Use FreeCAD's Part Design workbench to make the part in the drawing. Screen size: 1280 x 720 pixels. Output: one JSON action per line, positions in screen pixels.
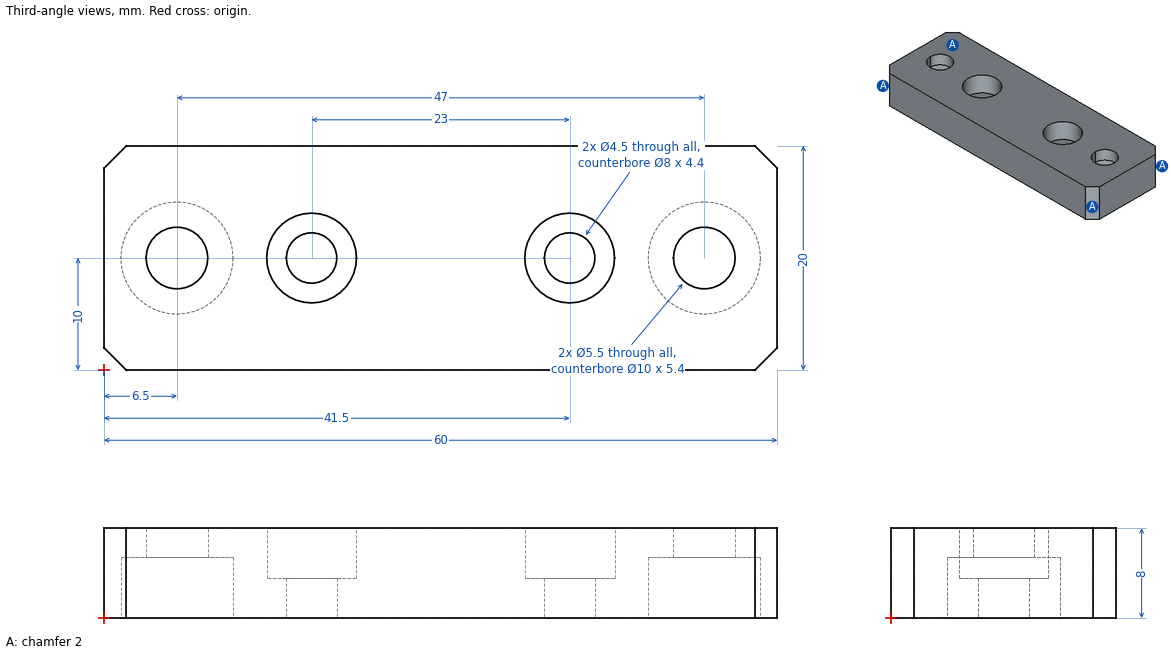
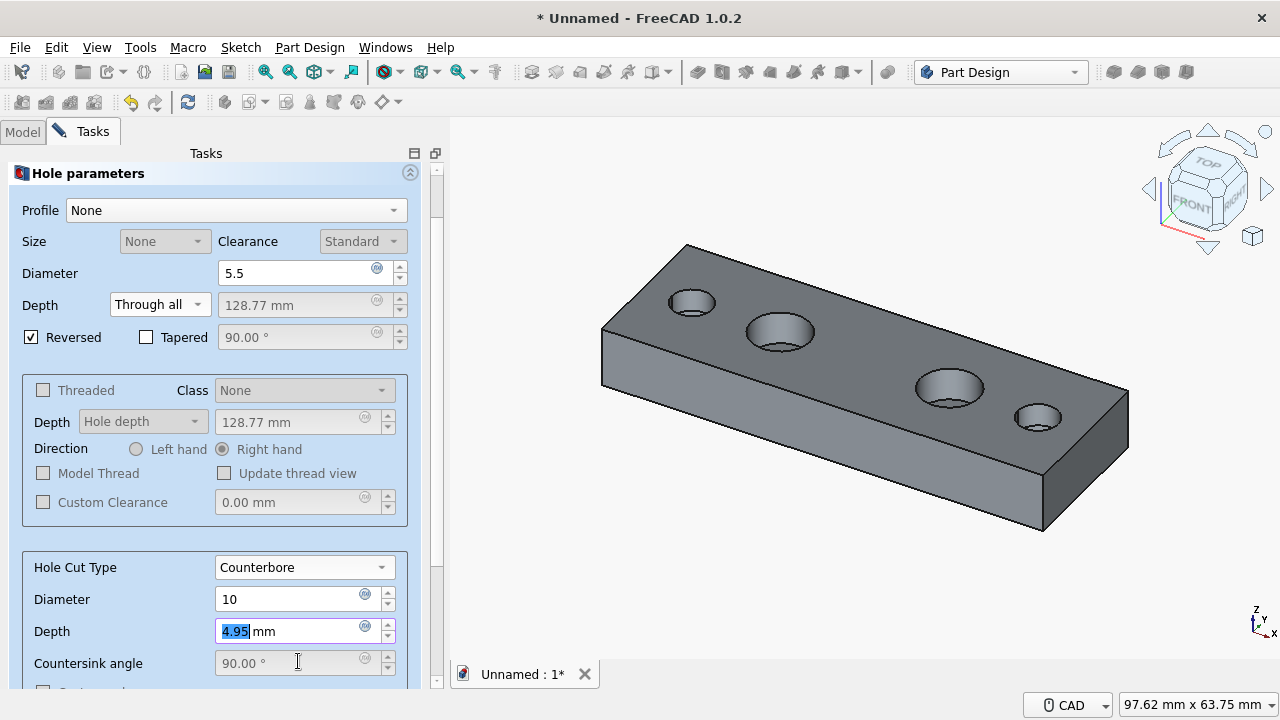
{"action": "type", "text": "5.4"}
{"action": "key", "text": "Tab"}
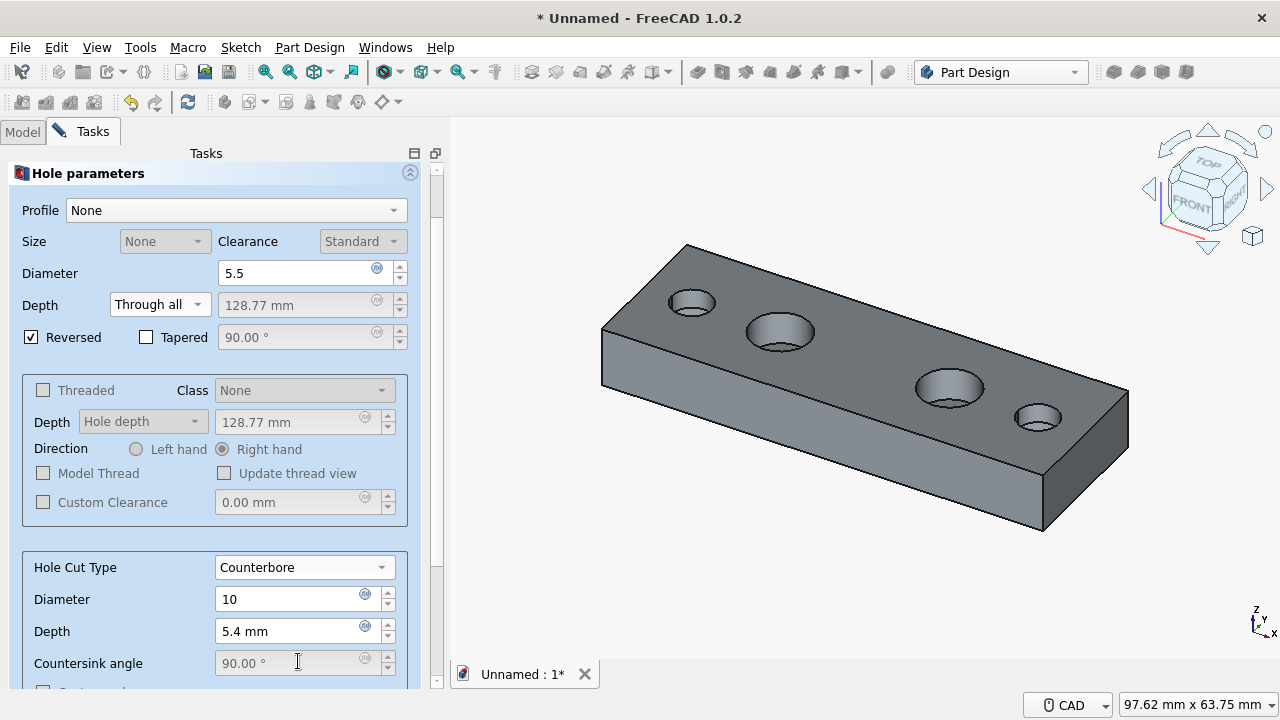
{"action": "scroll", "coordinate": [437, 426], "scroll_direction": "up", "scroll_amount": 2}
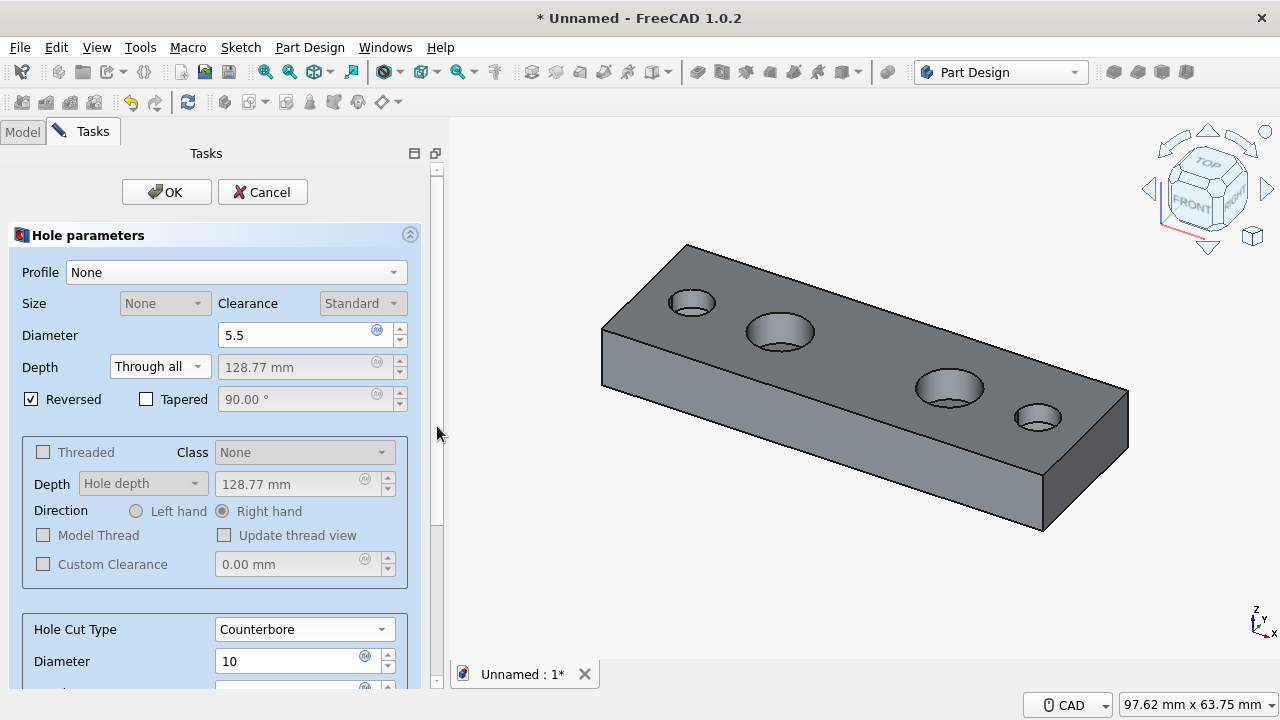
{"action": "left_click", "coordinate": [167, 192]}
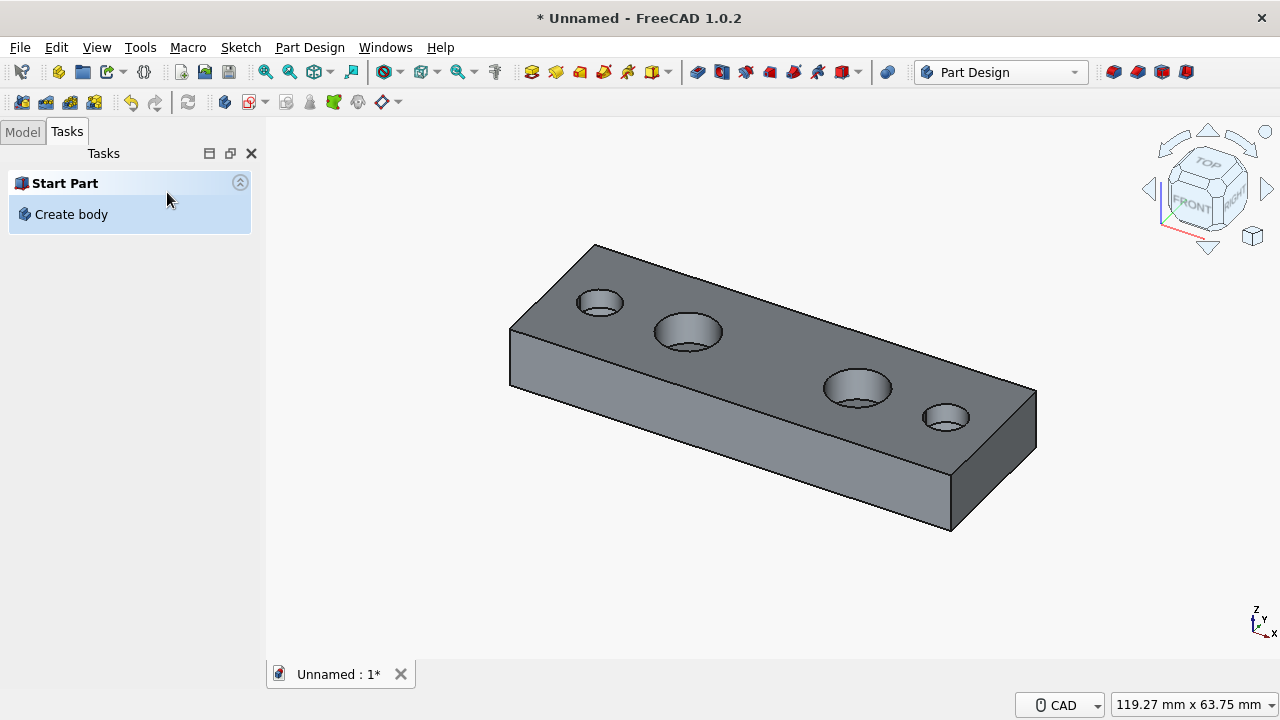
{"action": "left_click", "coordinate": [951, 502]}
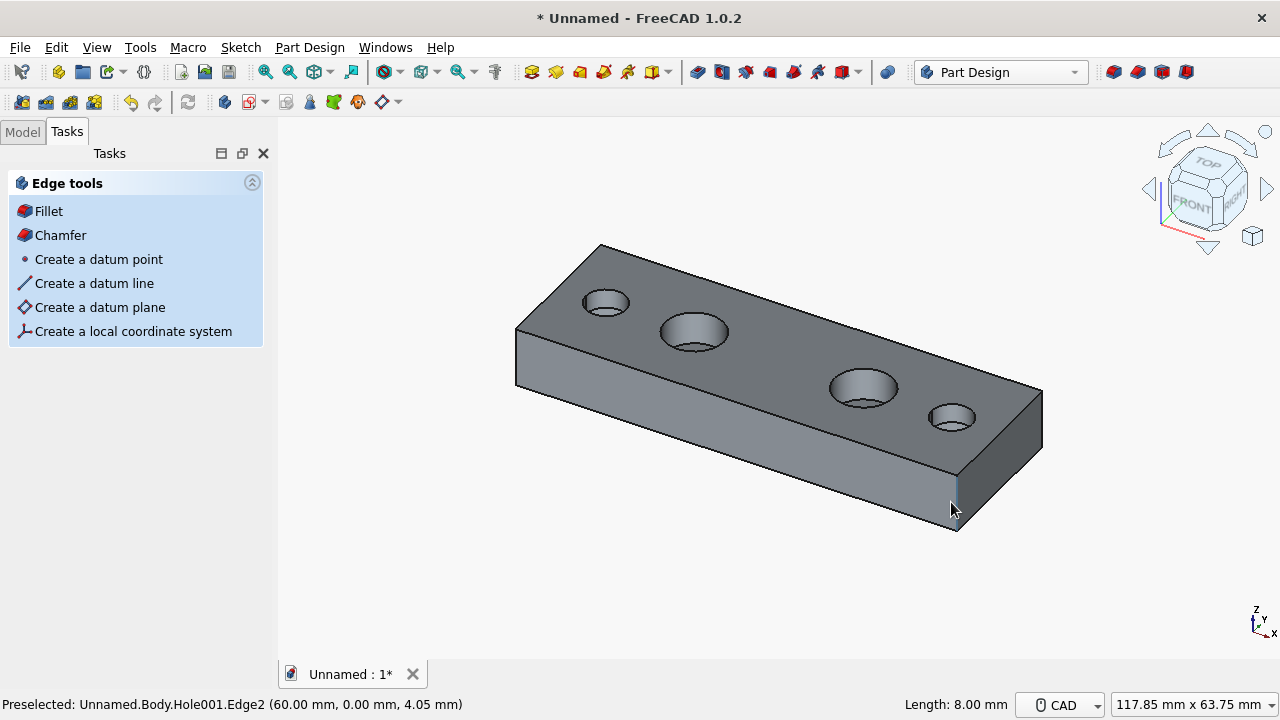
{"action": "key", "text": "0"}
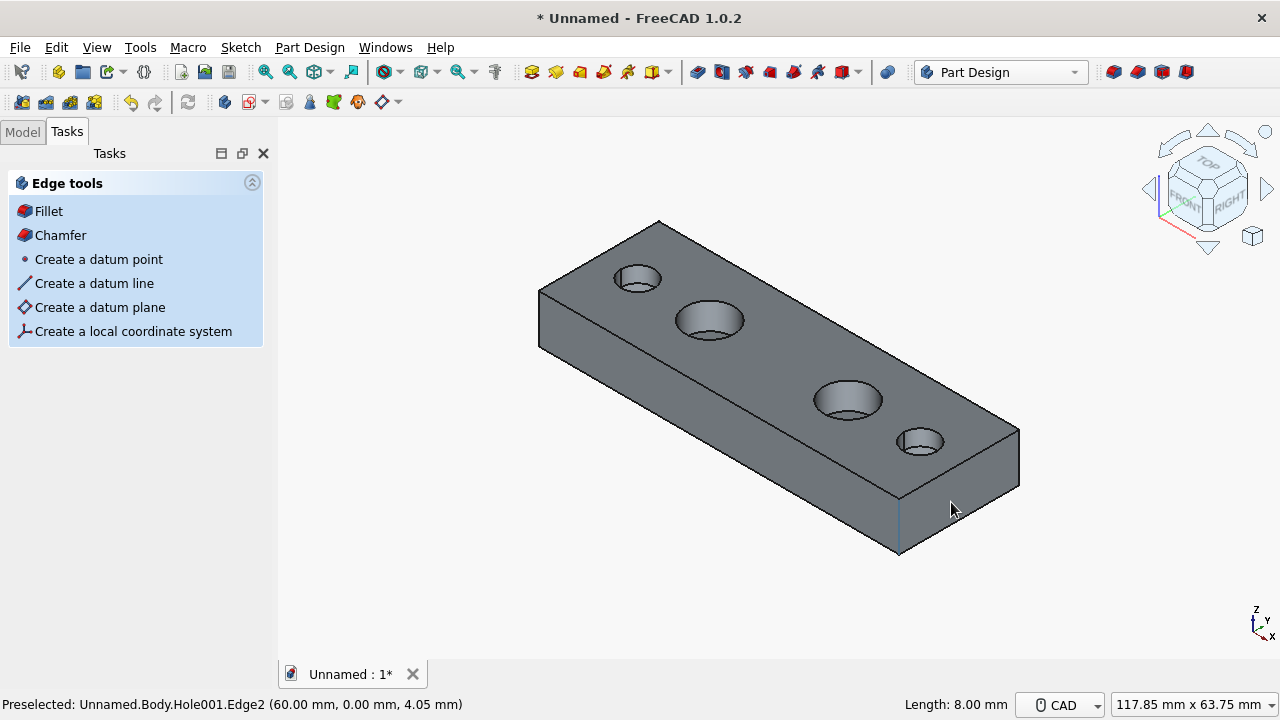
{"action": "key", "text": "2"}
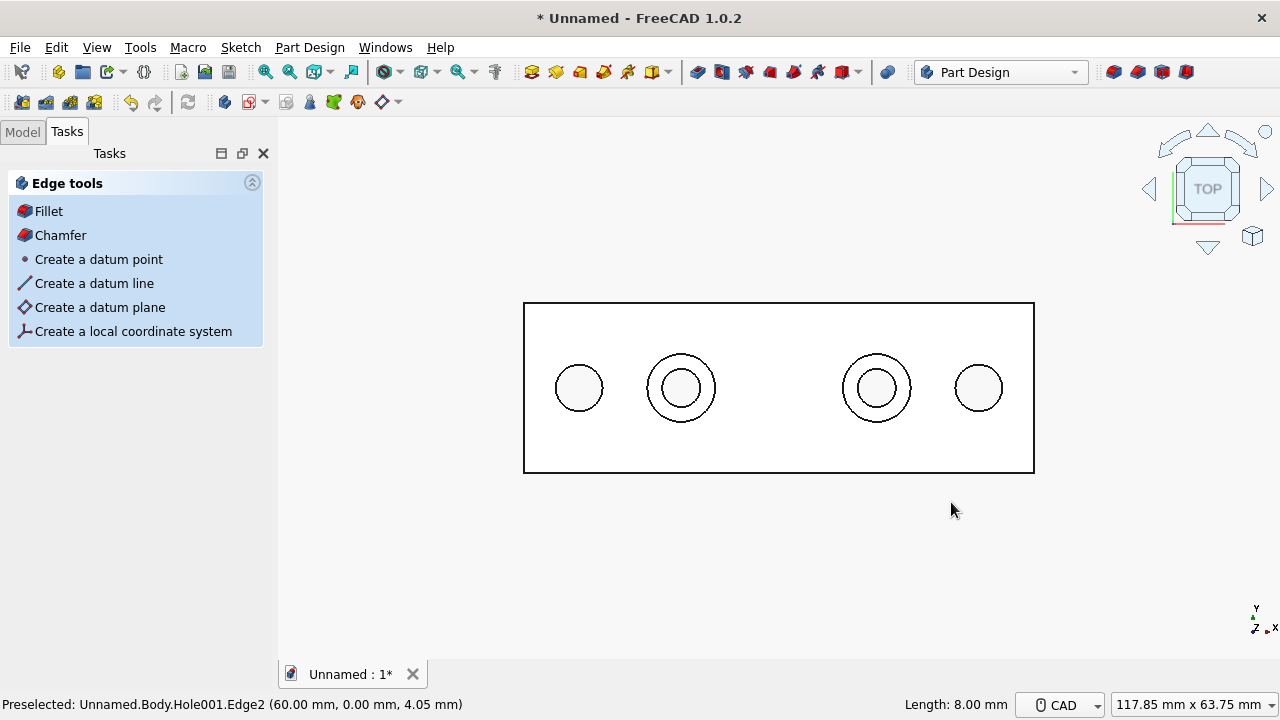
{"action": "key", "text": "1"}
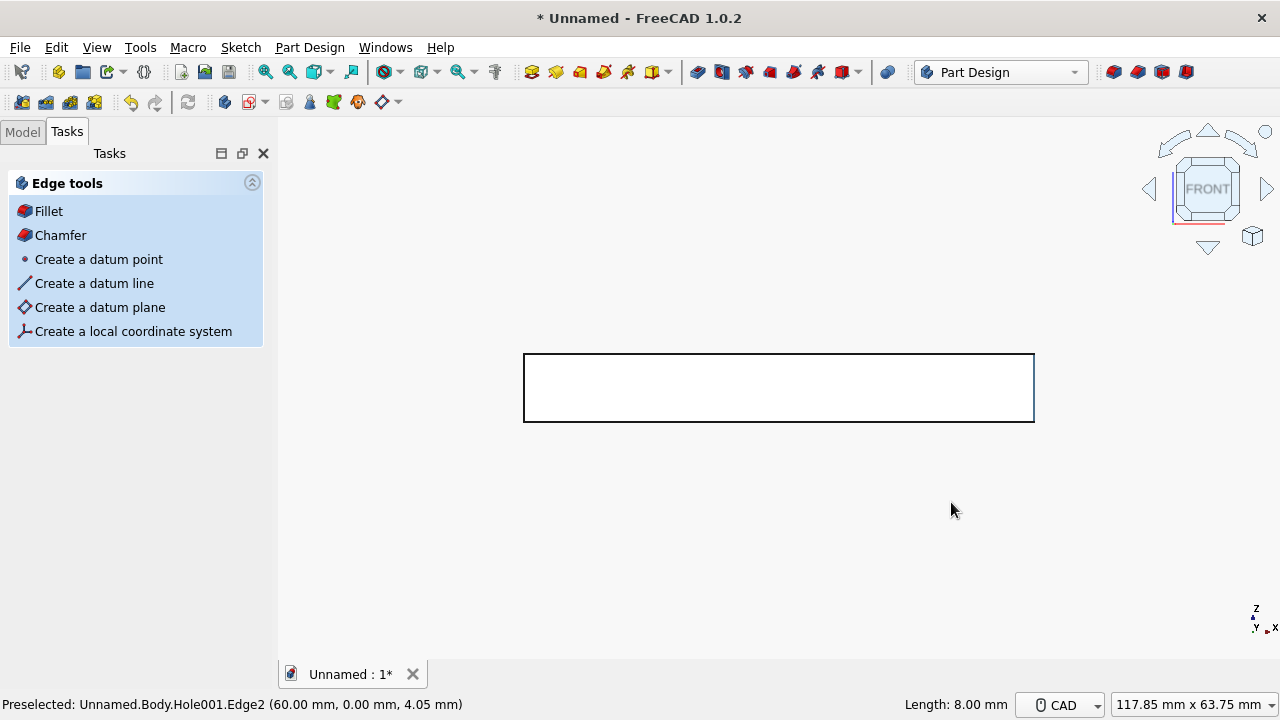
{"action": "left_click", "coordinate": [524, 387], "text": "ctrl"}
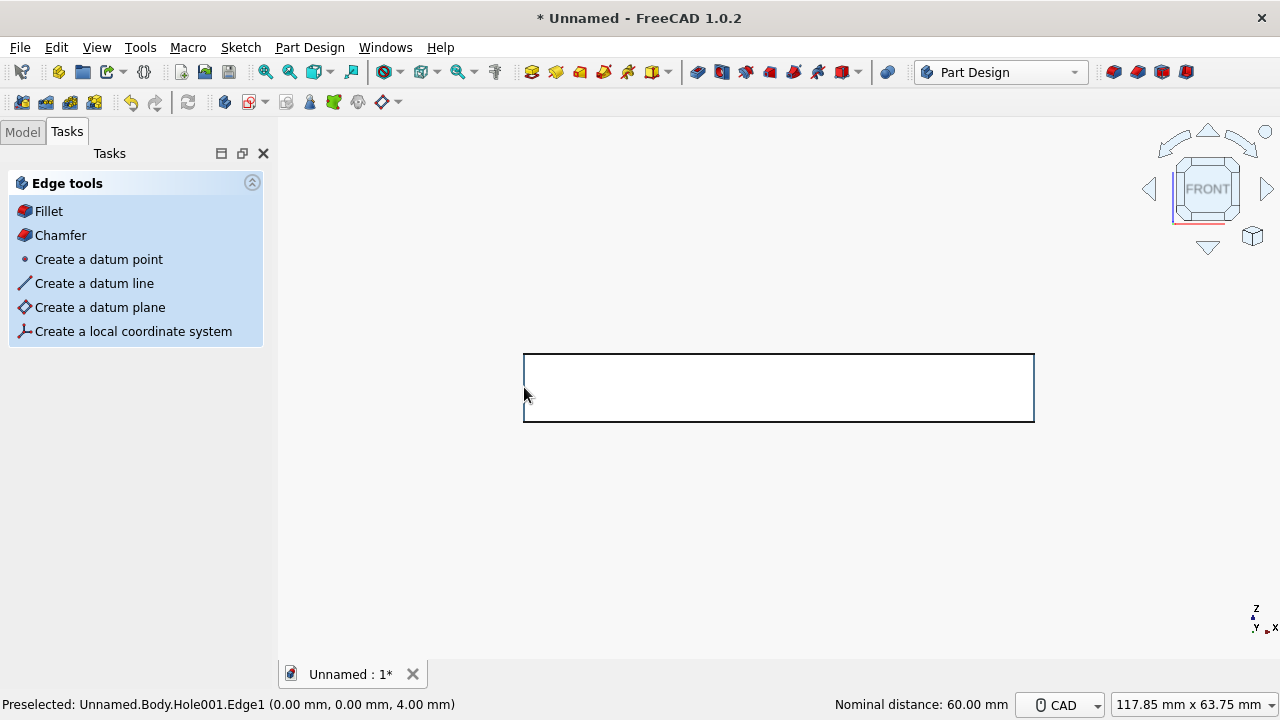
{"action": "key", "text": "3"}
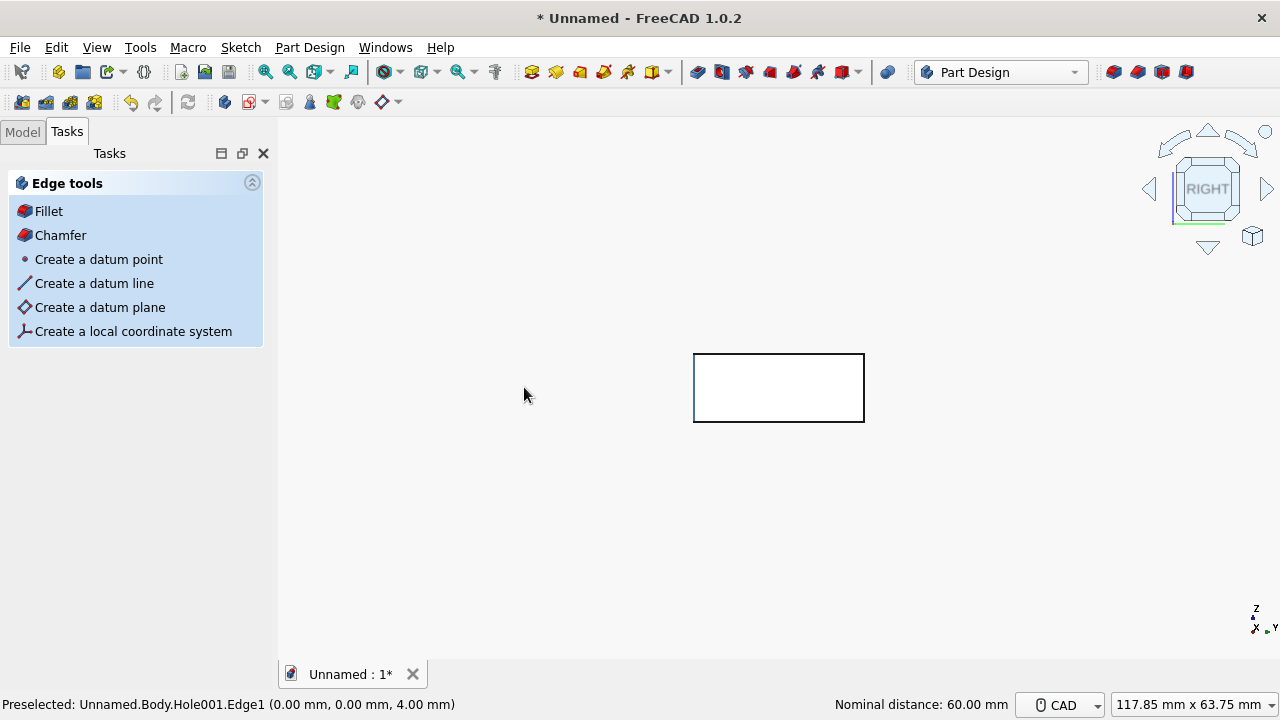
{"action": "key", "text": "v f"}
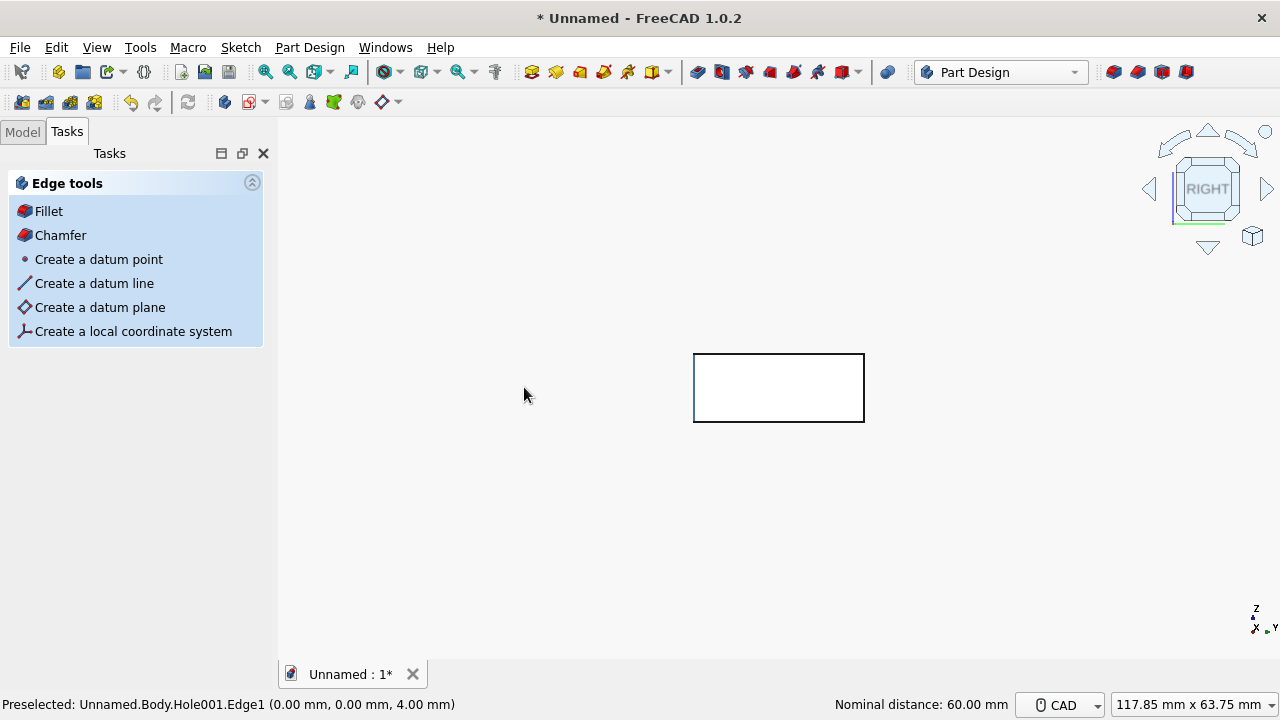
{"action": "left_click", "coordinate": [864, 387], "text": "ctrl"}